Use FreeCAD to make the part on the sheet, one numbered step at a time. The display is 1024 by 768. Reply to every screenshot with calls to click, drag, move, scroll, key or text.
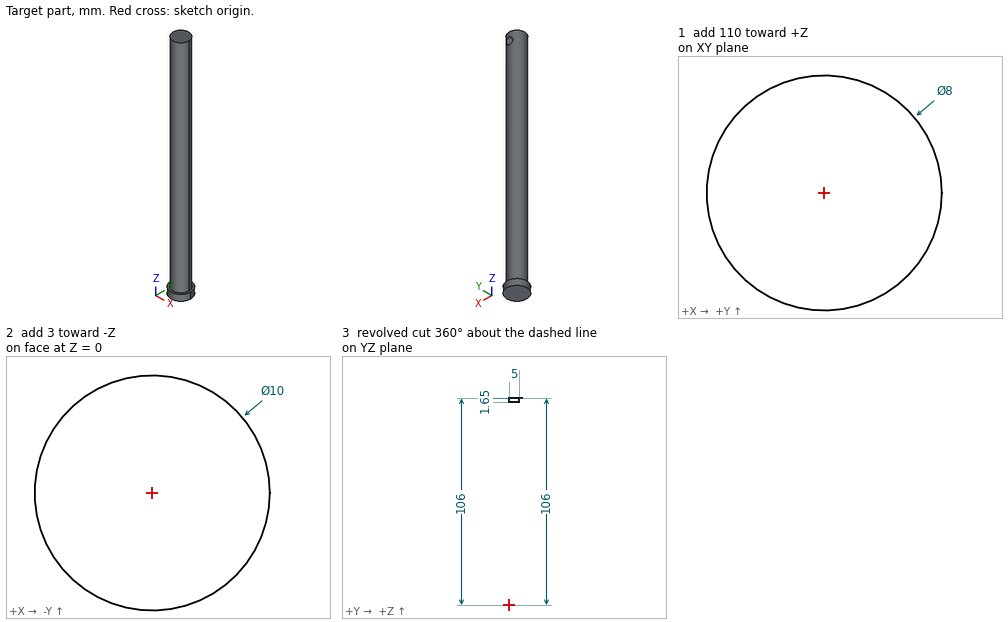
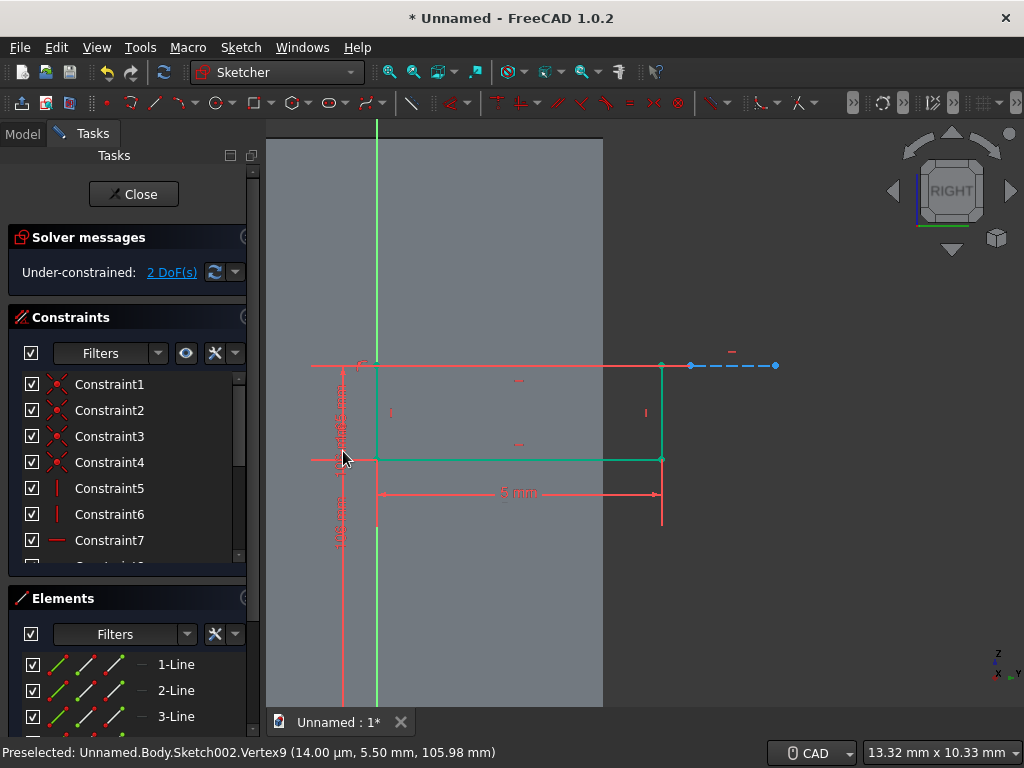
click(134, 194)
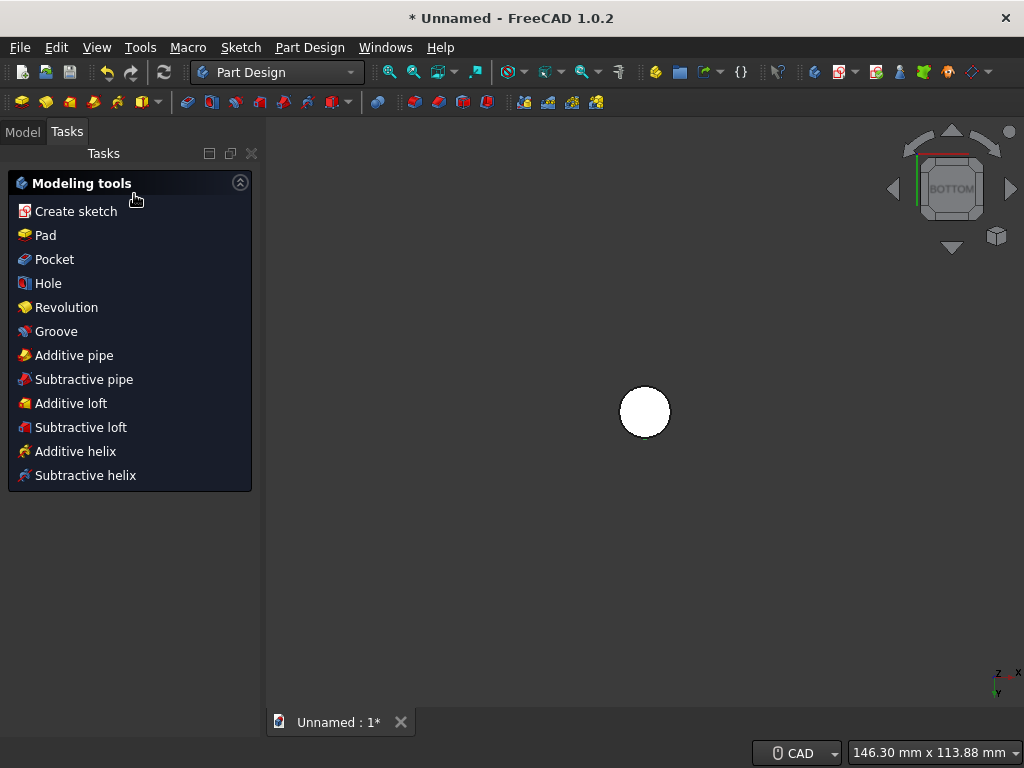
click(236, 102)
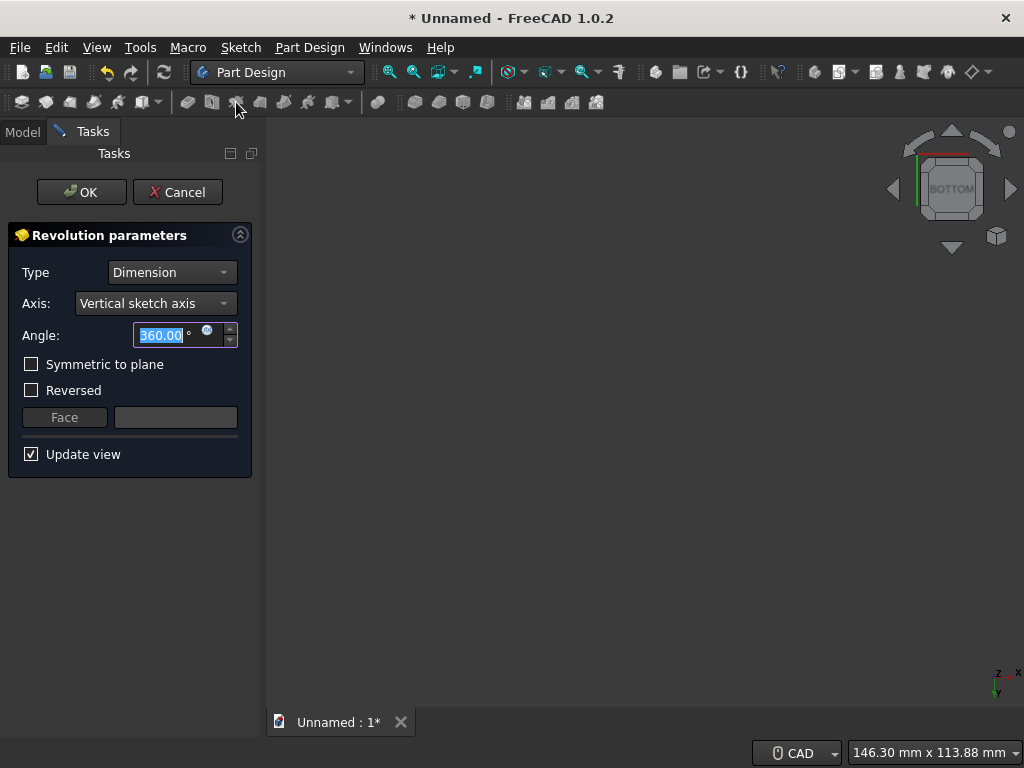
click(156, 304)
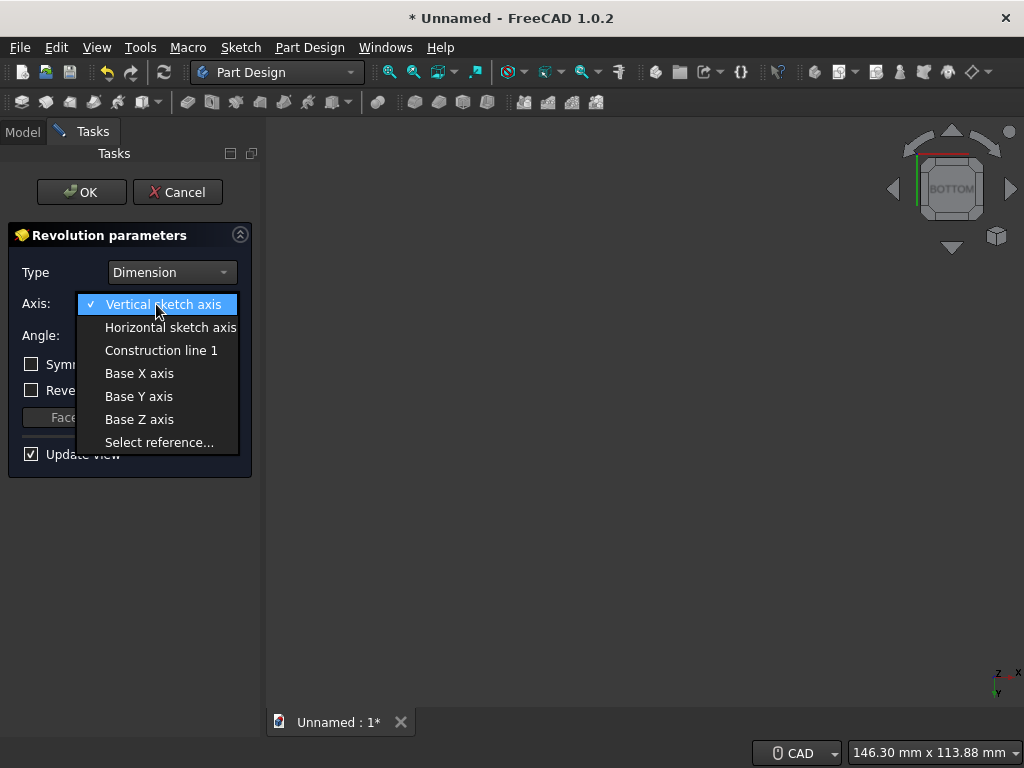
click(156, 350)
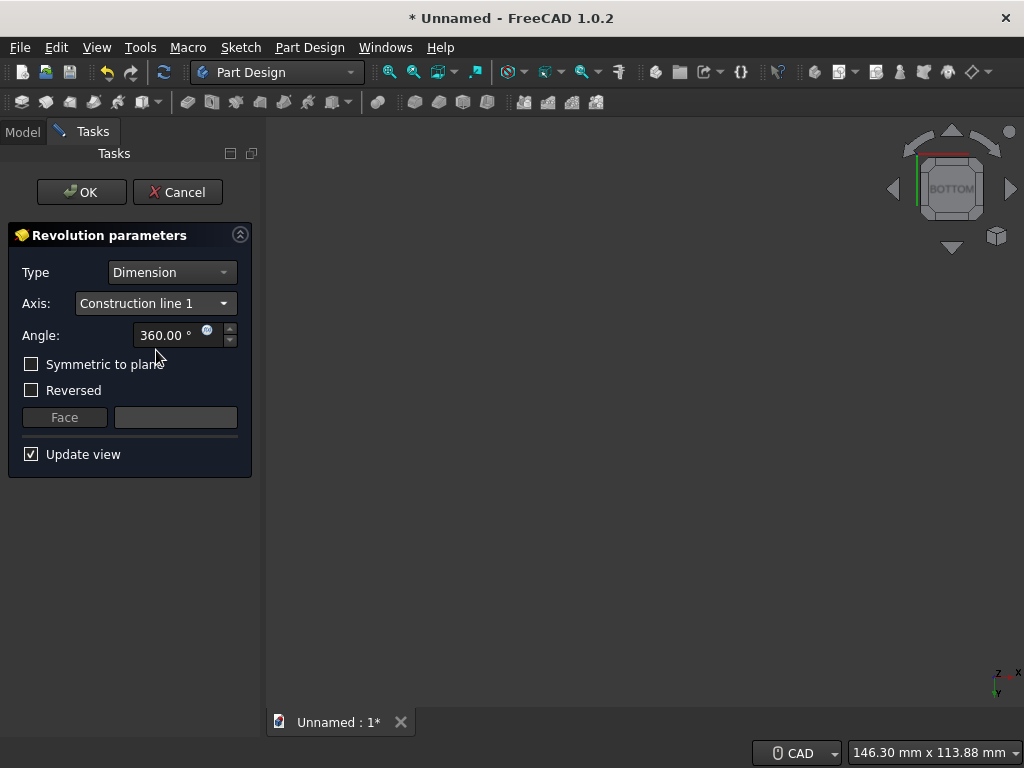
click(82, 192)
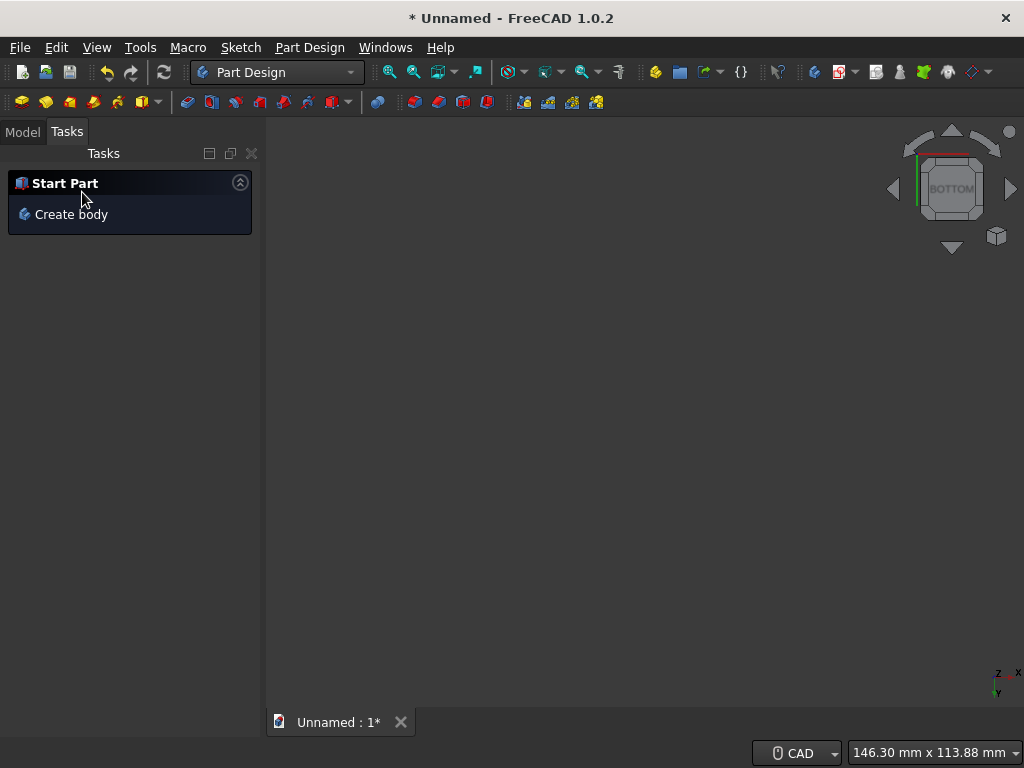
key(0)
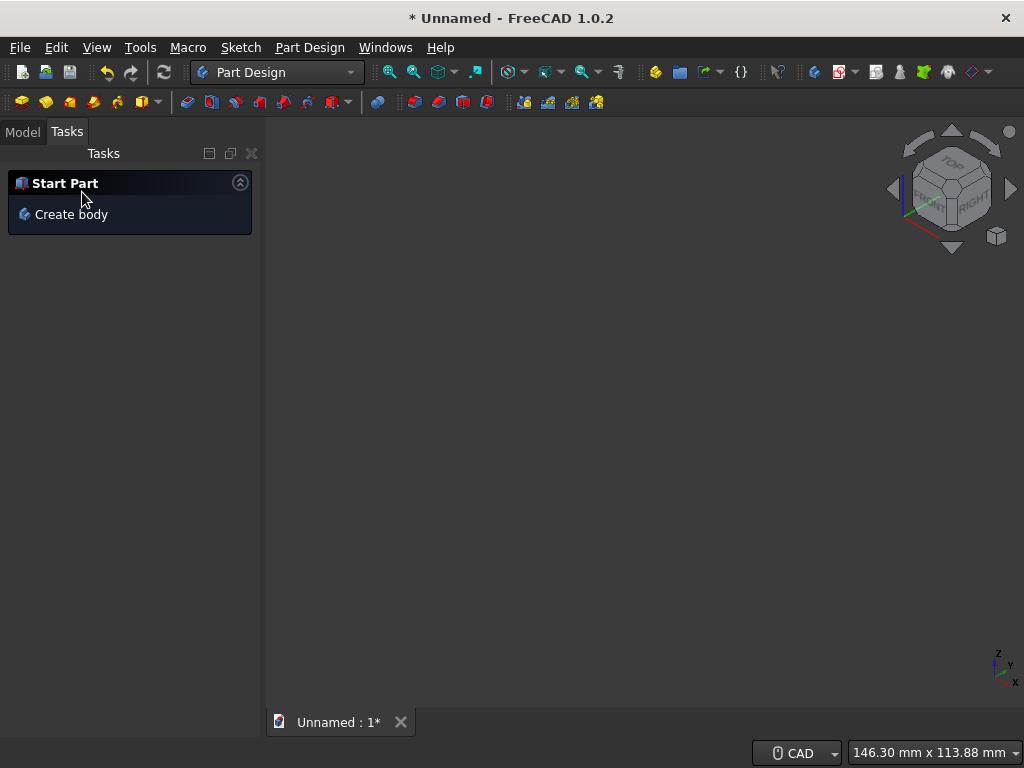
click(390, 72)